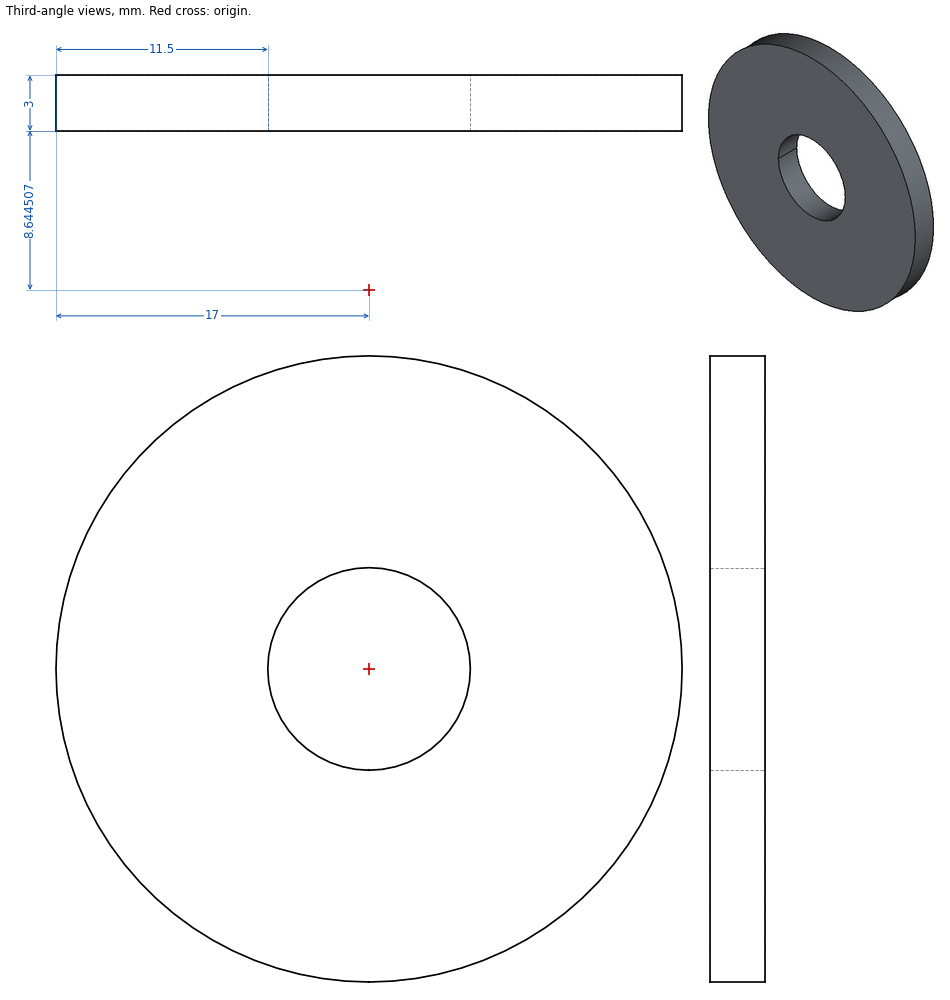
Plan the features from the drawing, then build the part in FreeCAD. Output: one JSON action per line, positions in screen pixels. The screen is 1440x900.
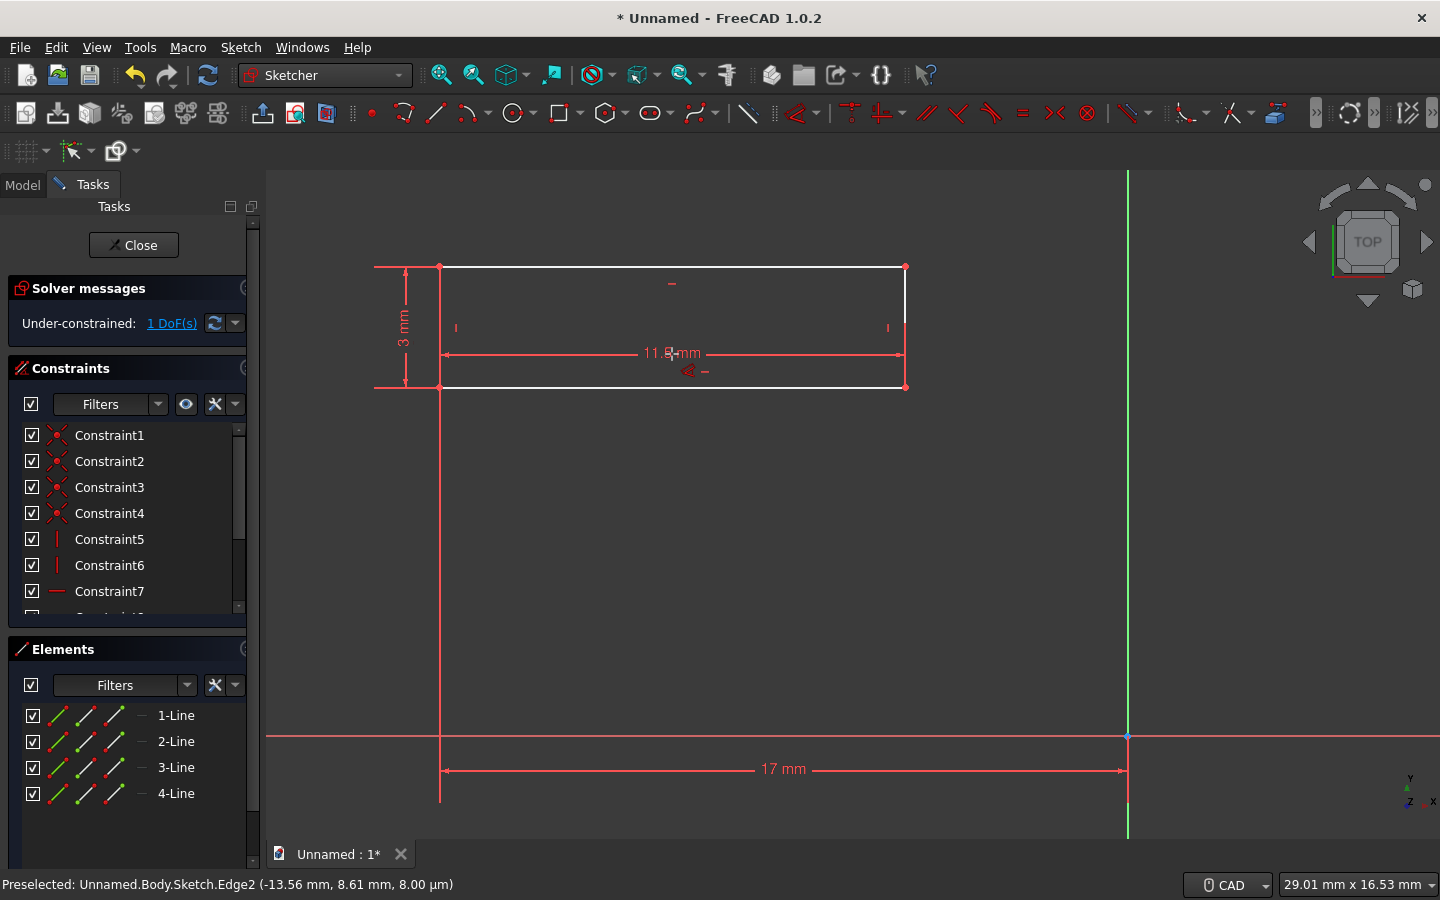
{"action": "left_click", "coordinate": [440, 388]}
{"action": "left_click", "coordinate": [1162, 562]}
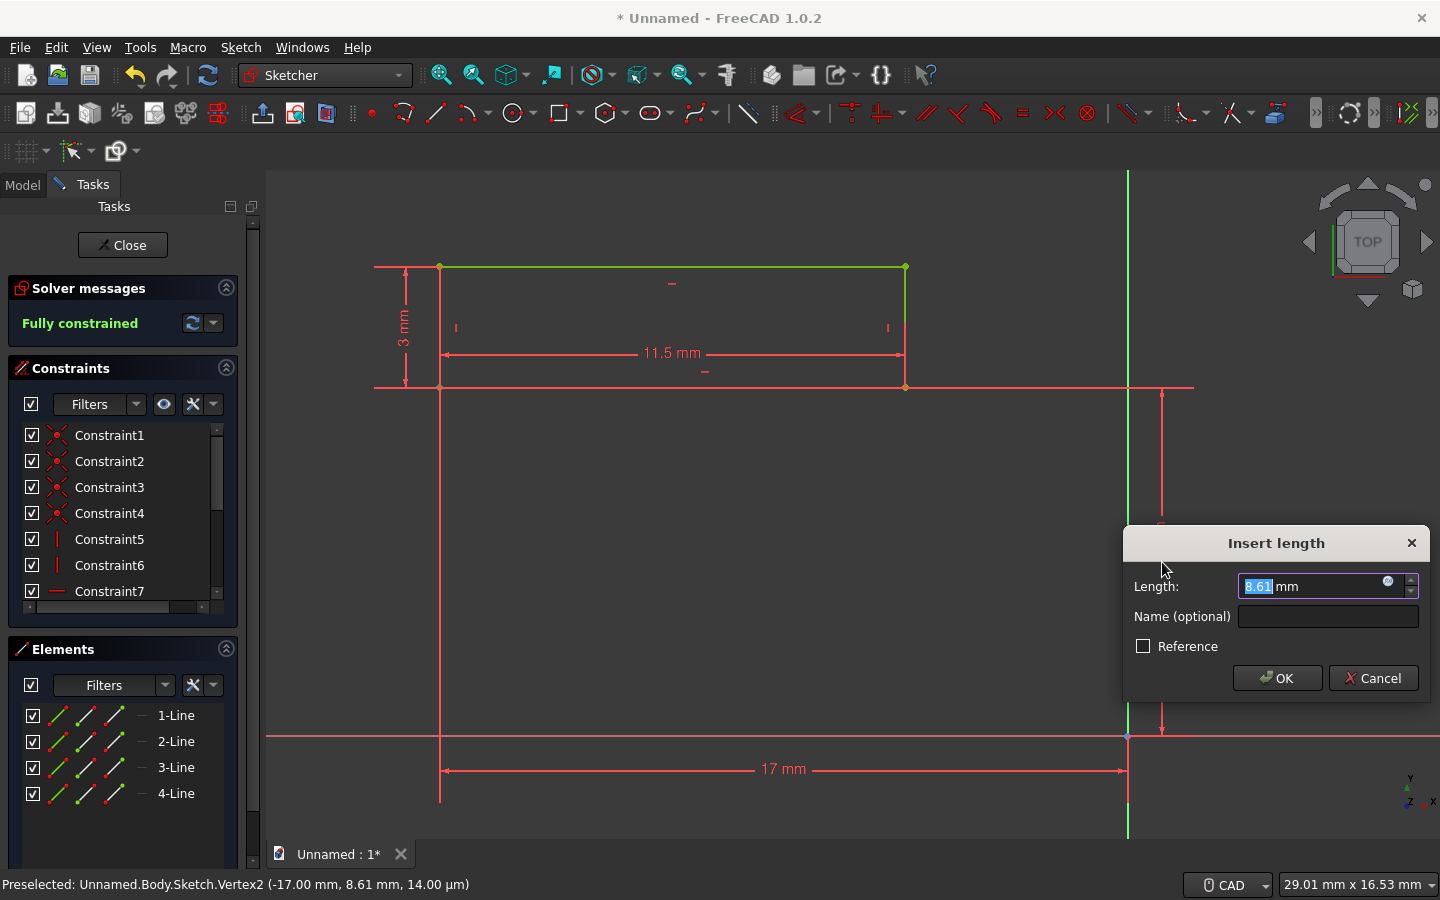
{"action": "type", "text": "8.644507"}
{"action": "key", "text": "Return"}
{"action": "key", "text": "Escape"}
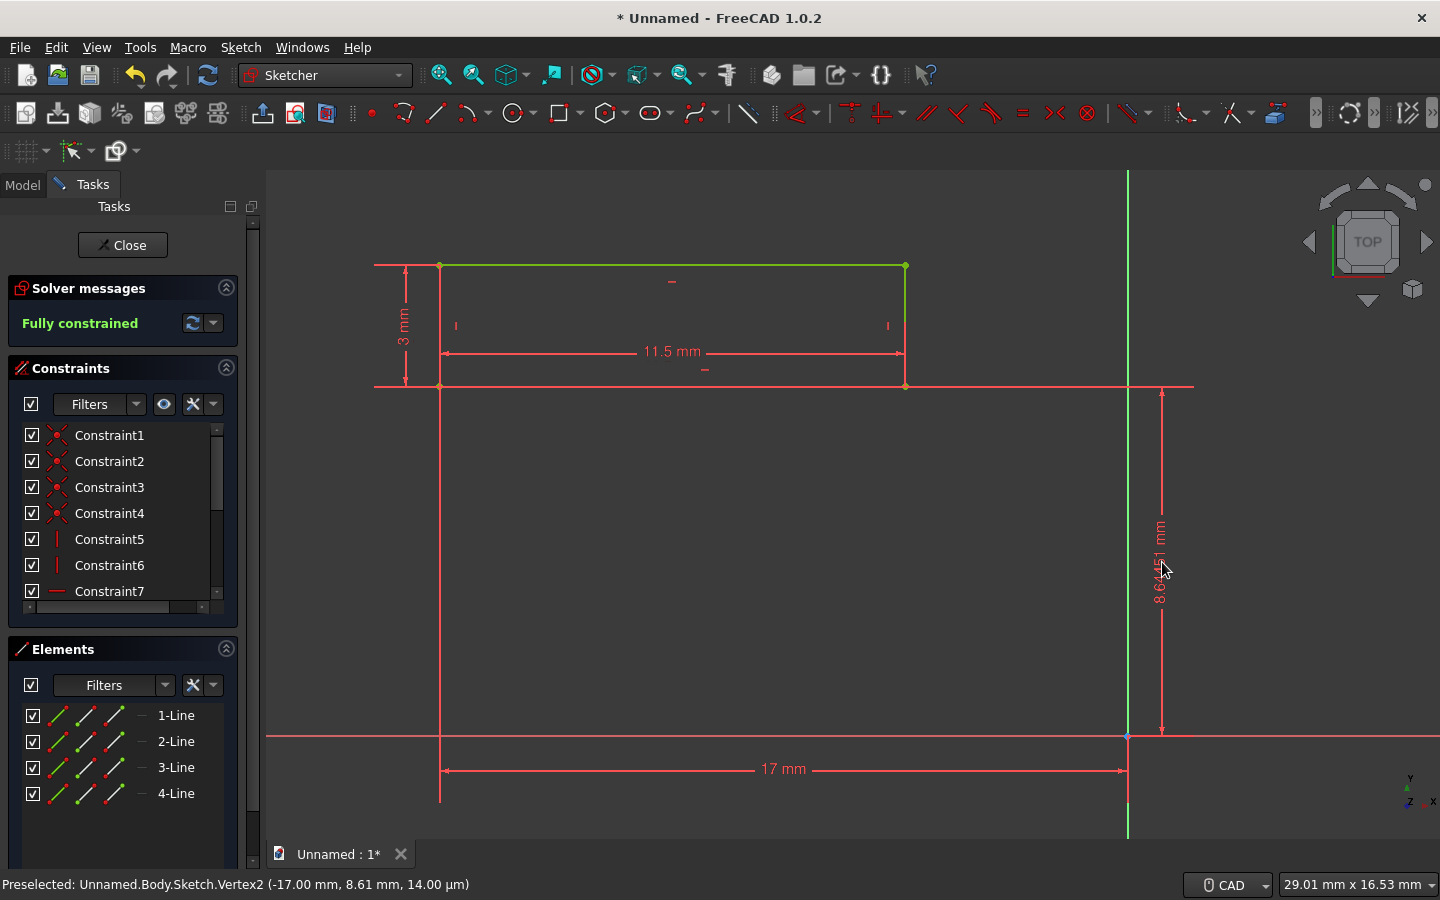
{"action": "left_click", "coordinate": [123, 245]}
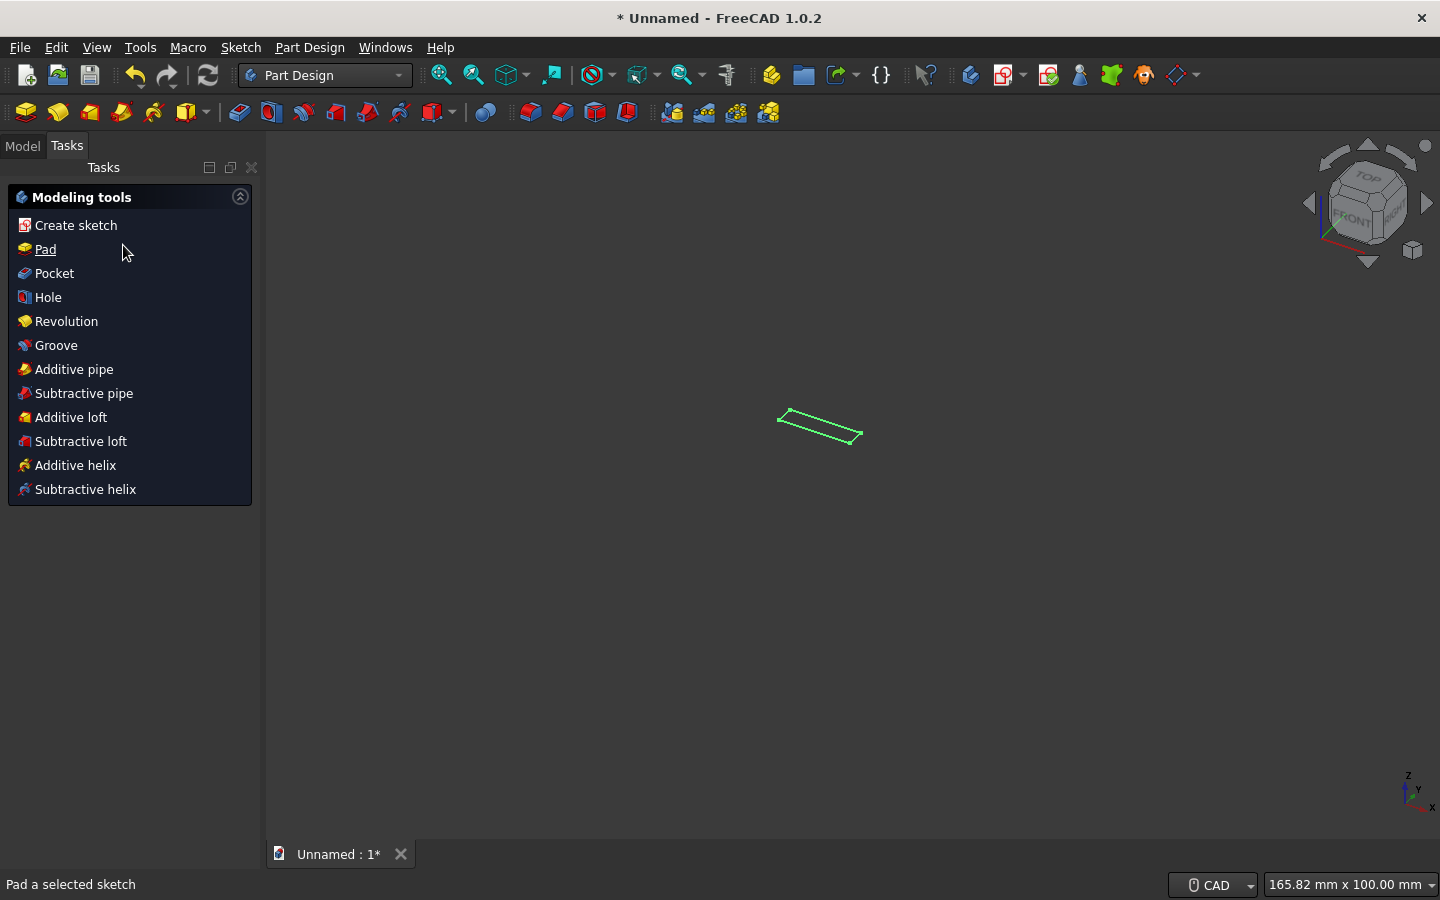
{"action": "left_click", "coordinate": [58, 112]}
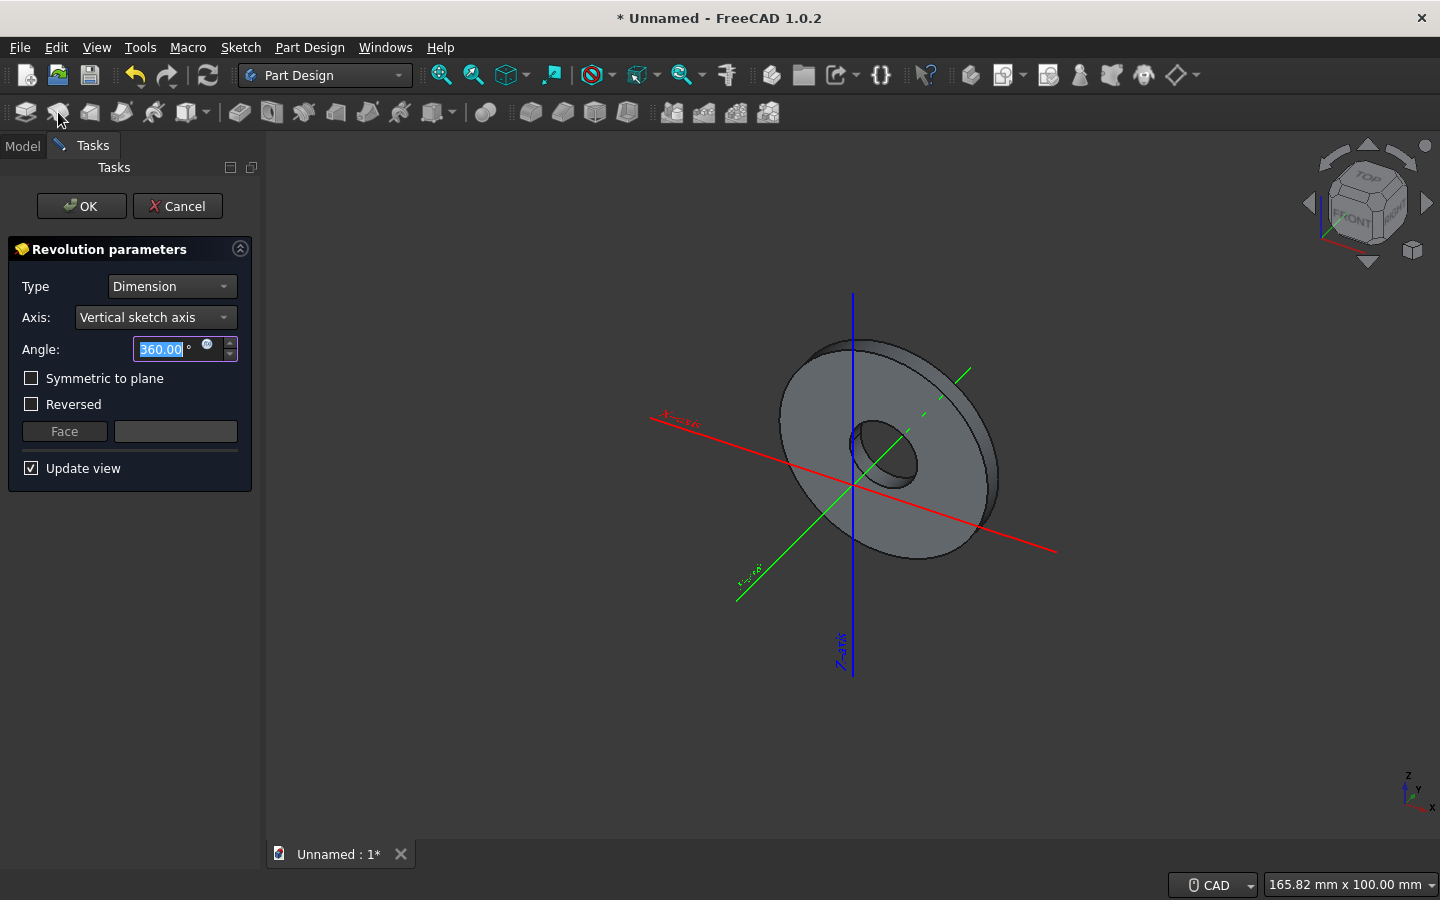
{"action": "left_click", "coordinate": [82, 206]}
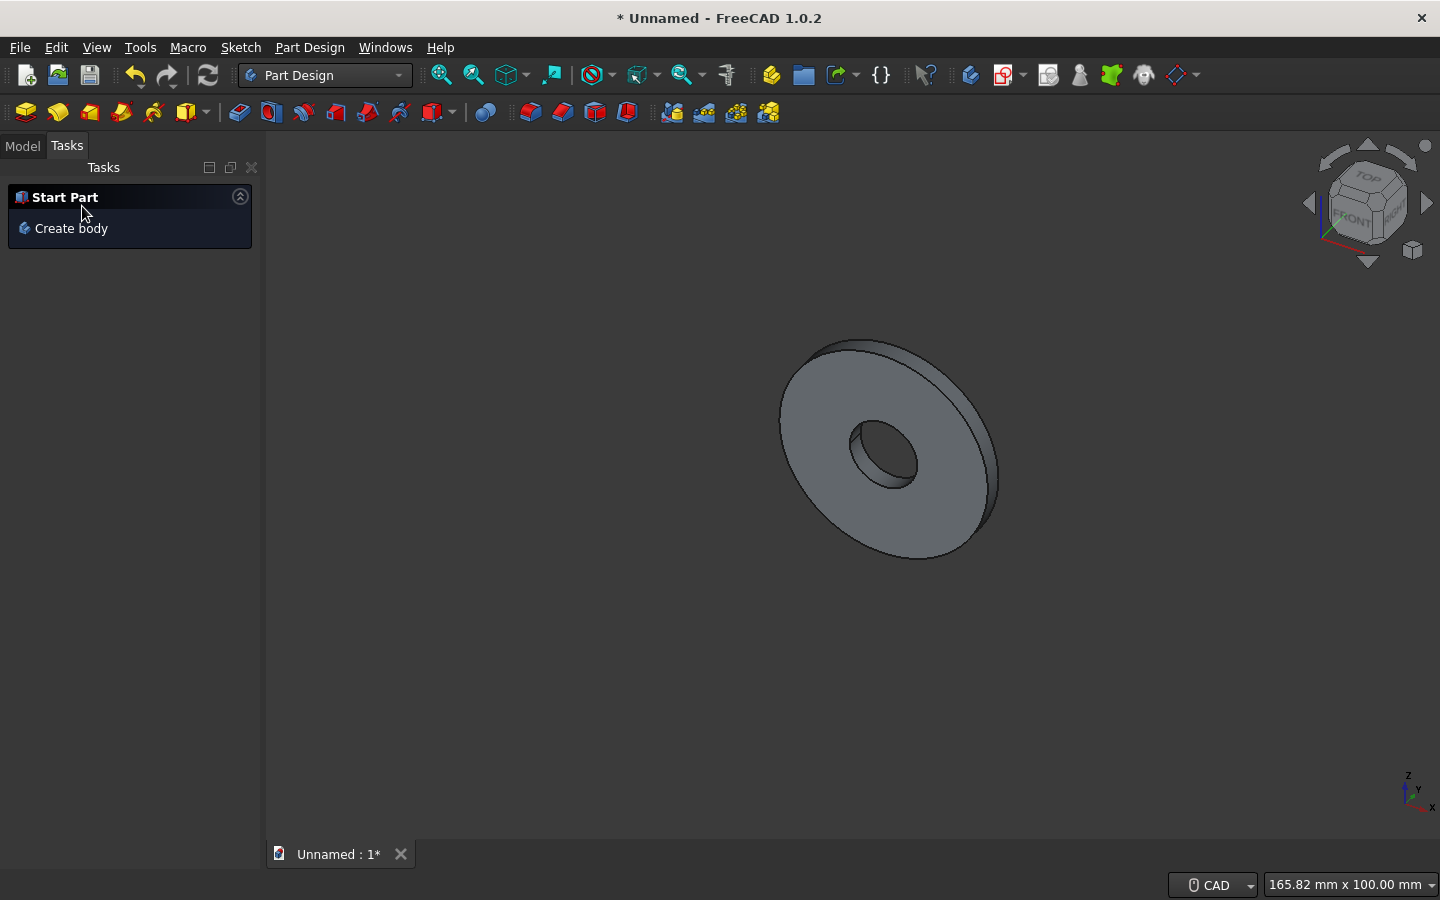
{"action": "key", "text": "0"}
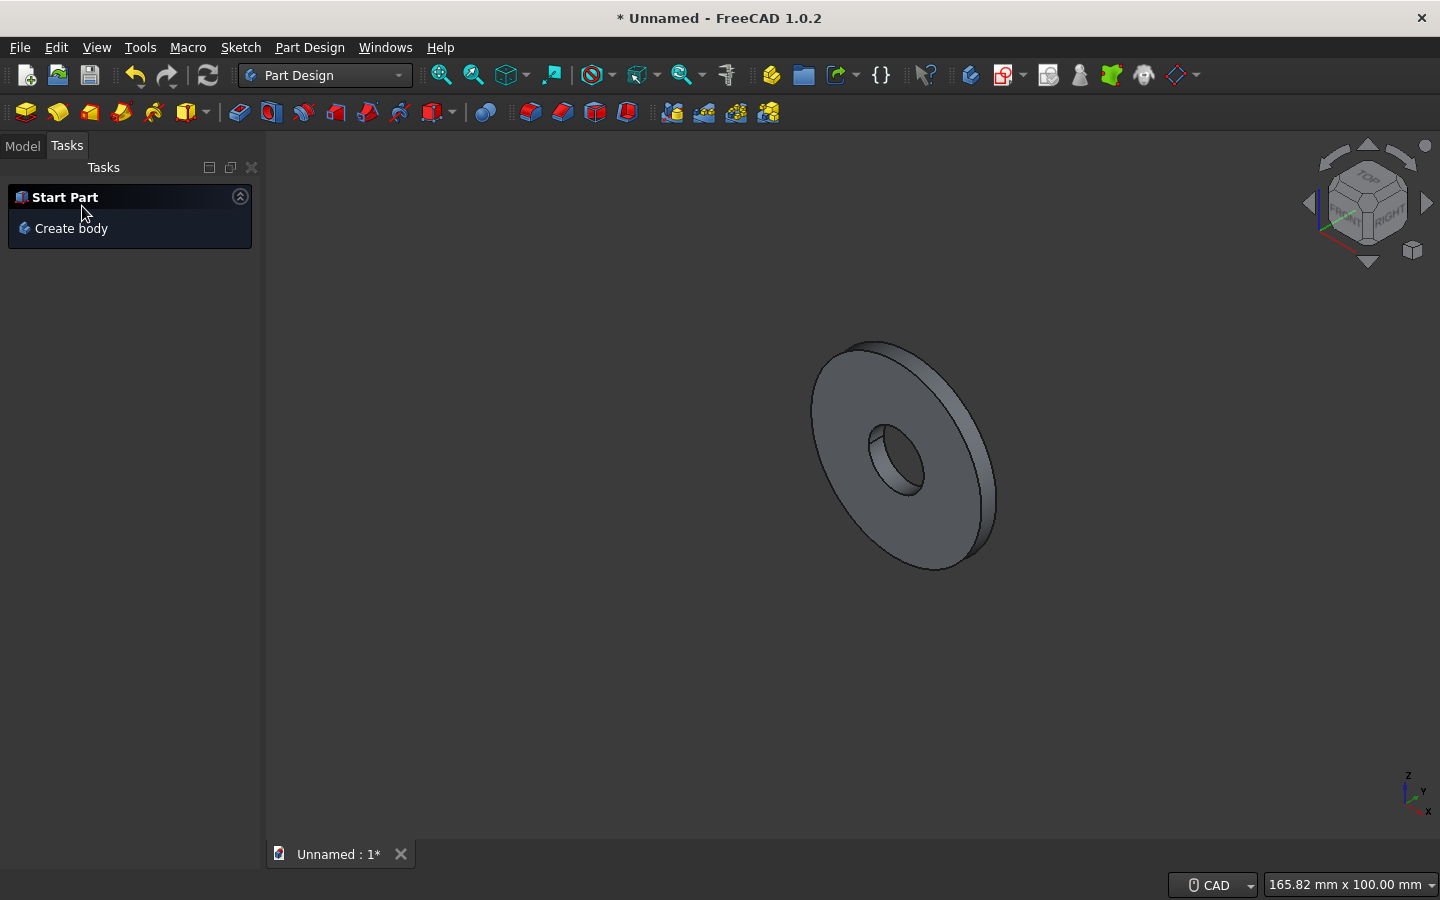
{"action": "left_click", "coordinate": [442, 76]}